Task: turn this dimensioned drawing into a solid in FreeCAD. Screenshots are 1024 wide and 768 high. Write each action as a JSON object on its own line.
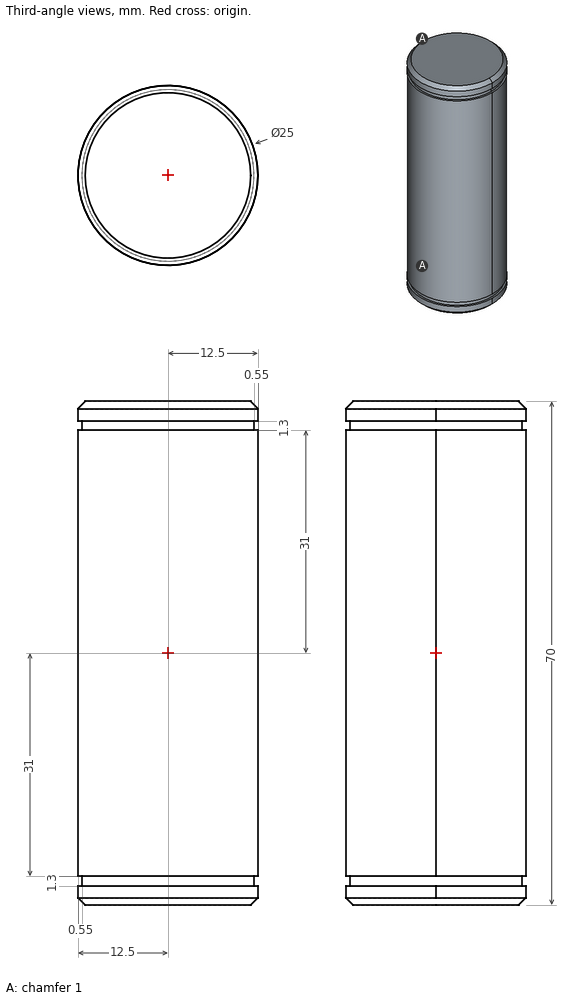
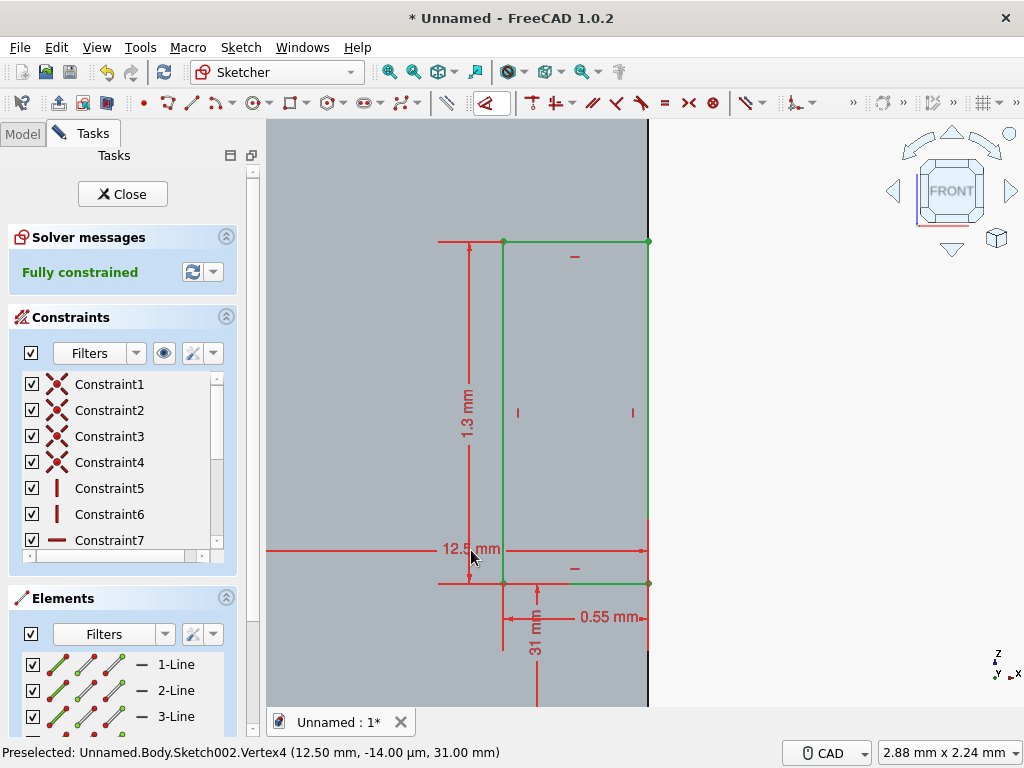
{"action": "left_click", "coordinate": [123, 194]}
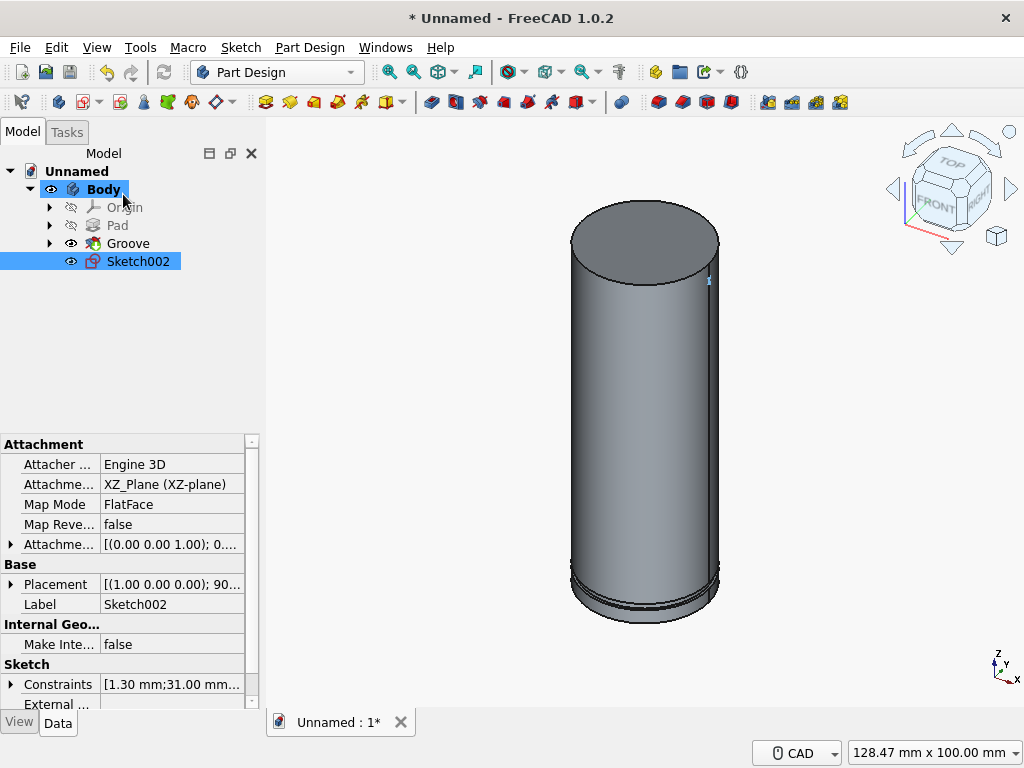
{"action": "left_click", "coordinate": [480, 102]}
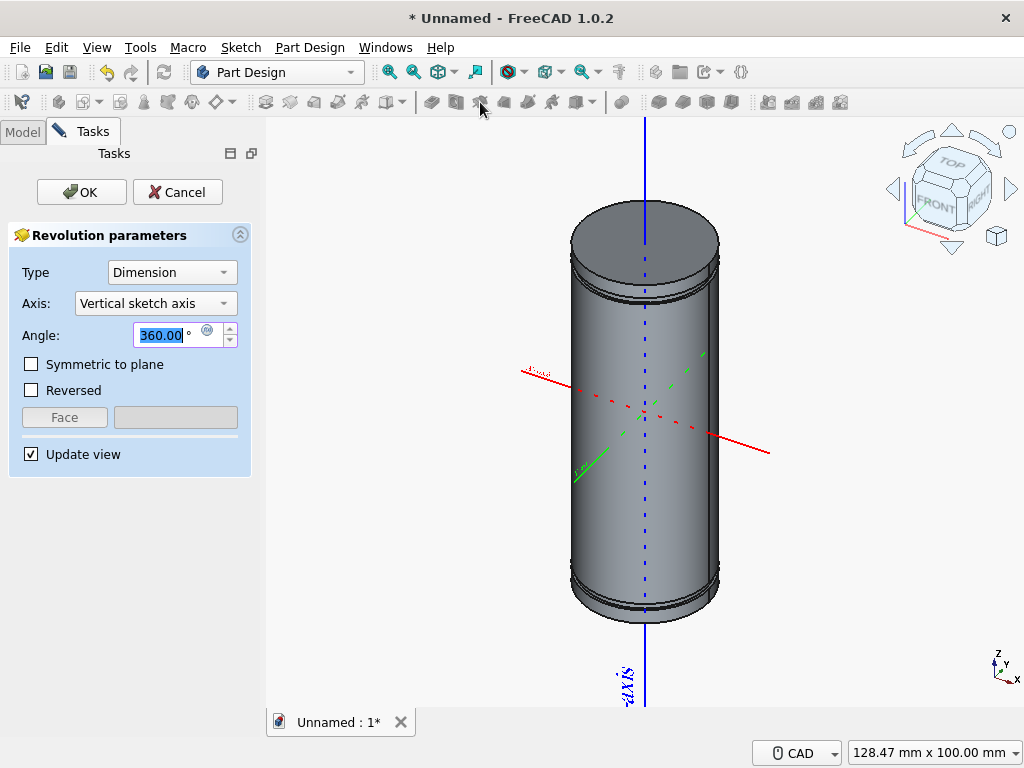
{"action": "left_click", "coordinate": [82, 192]}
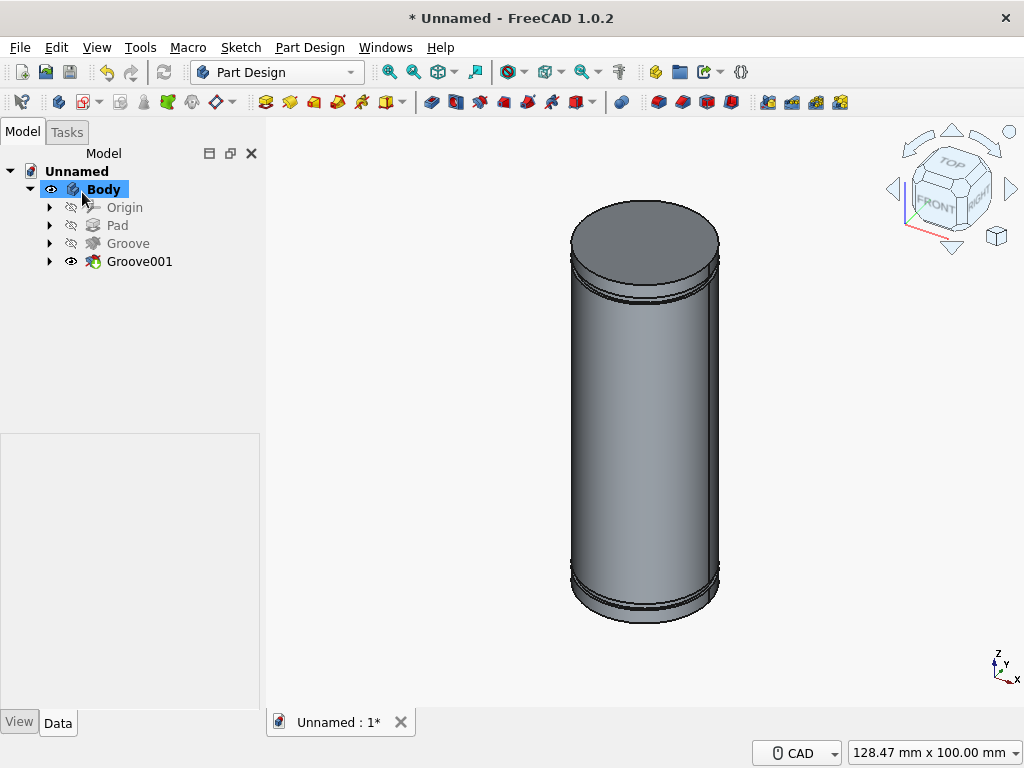
{"action": "left_click", "coordinate": [572, 246]}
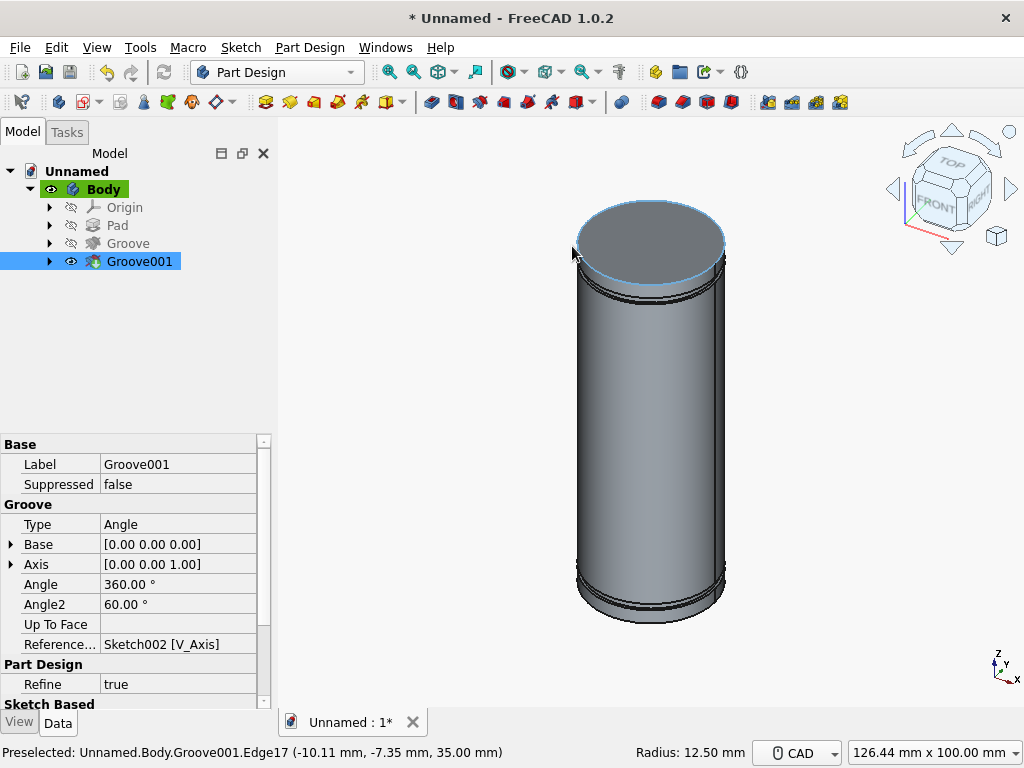
{"action": "key", "text": "0"}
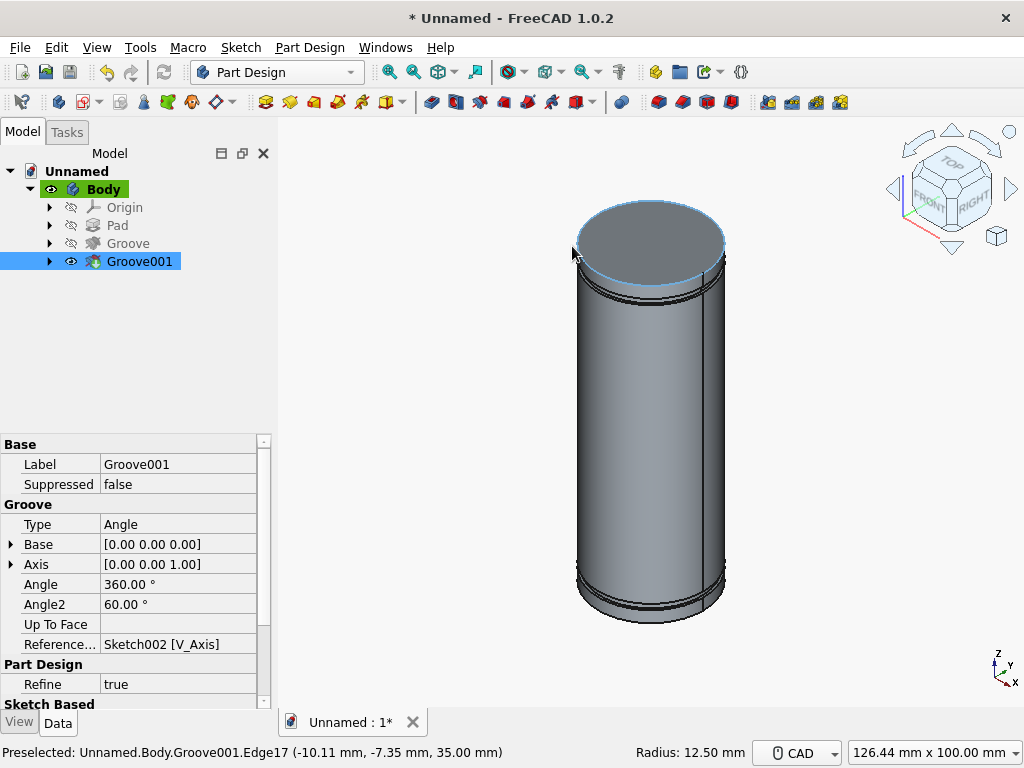
{"action": "key", "text": "2"}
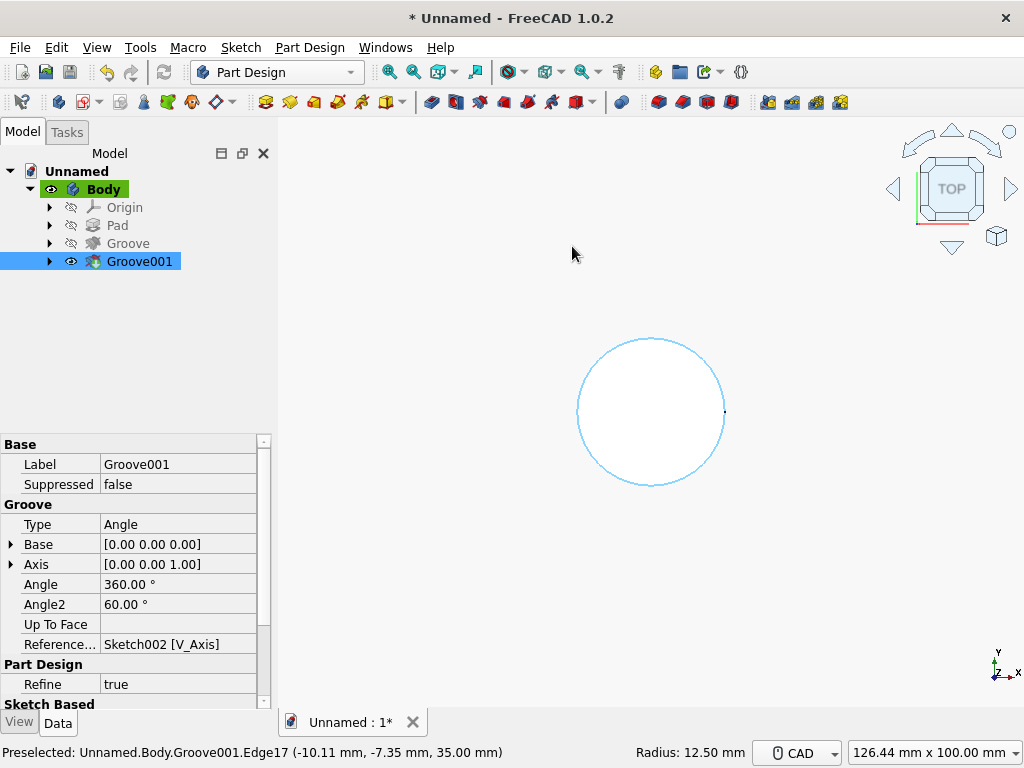
{"action": "key", "text": "v f"}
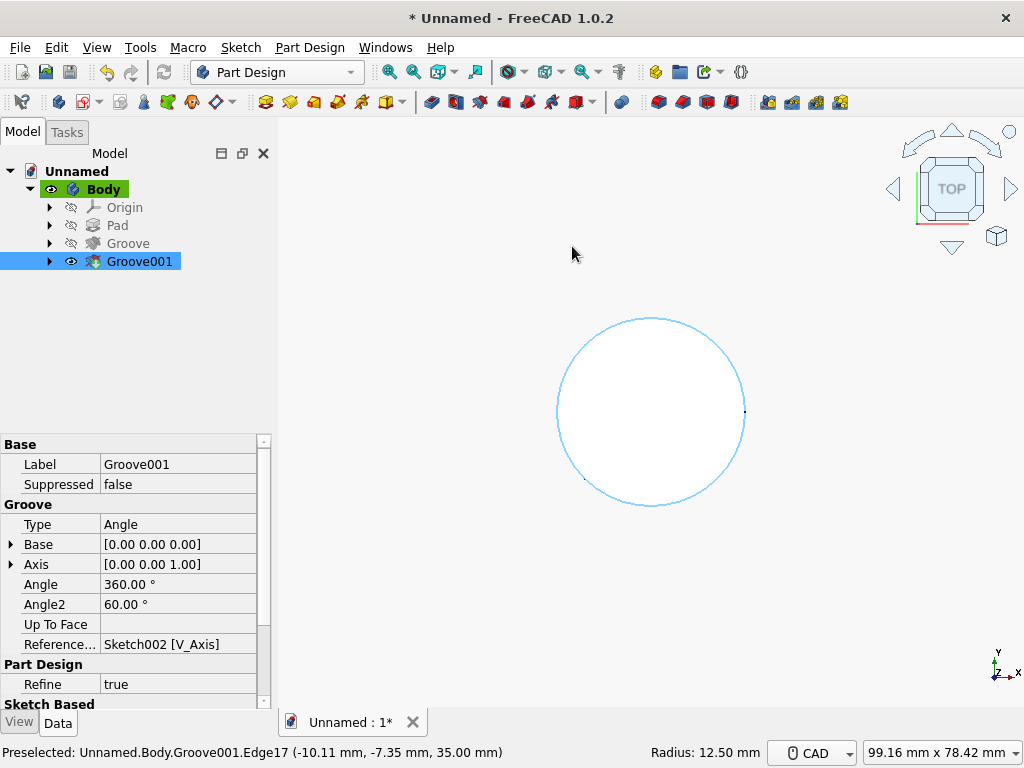
{"action": "key", "text": "1"}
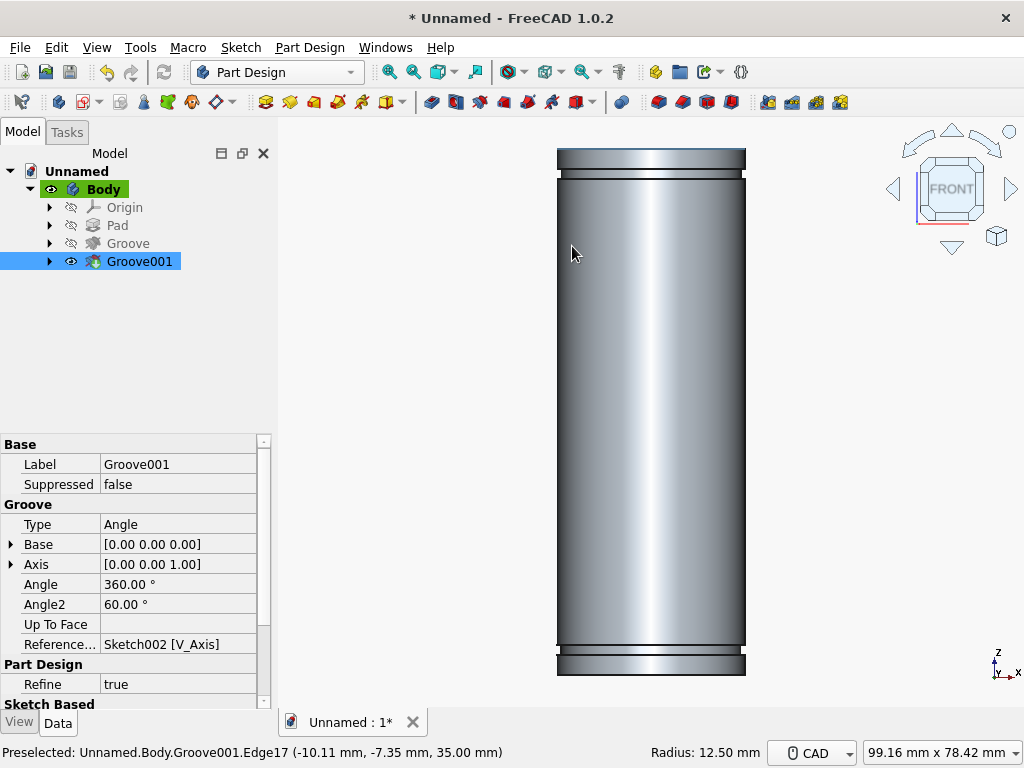
{"action": "left_click", "coordinate": [575, 674], "text": "ctrl"}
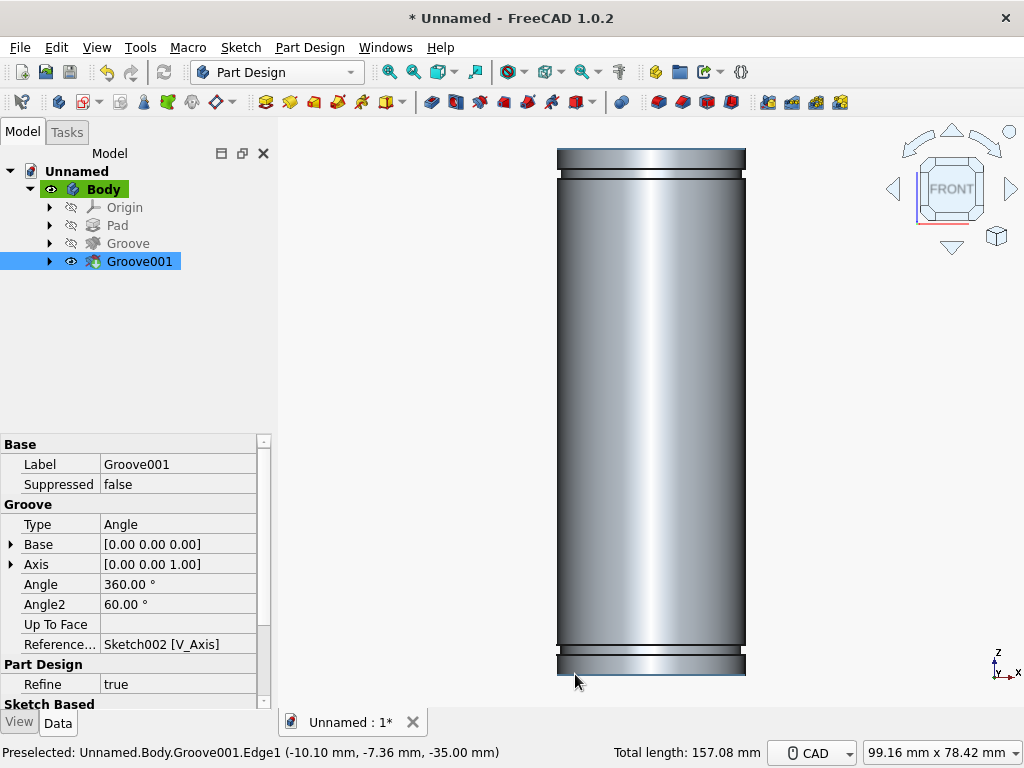
{"action": "left_click", "coordinate": [684, 102]}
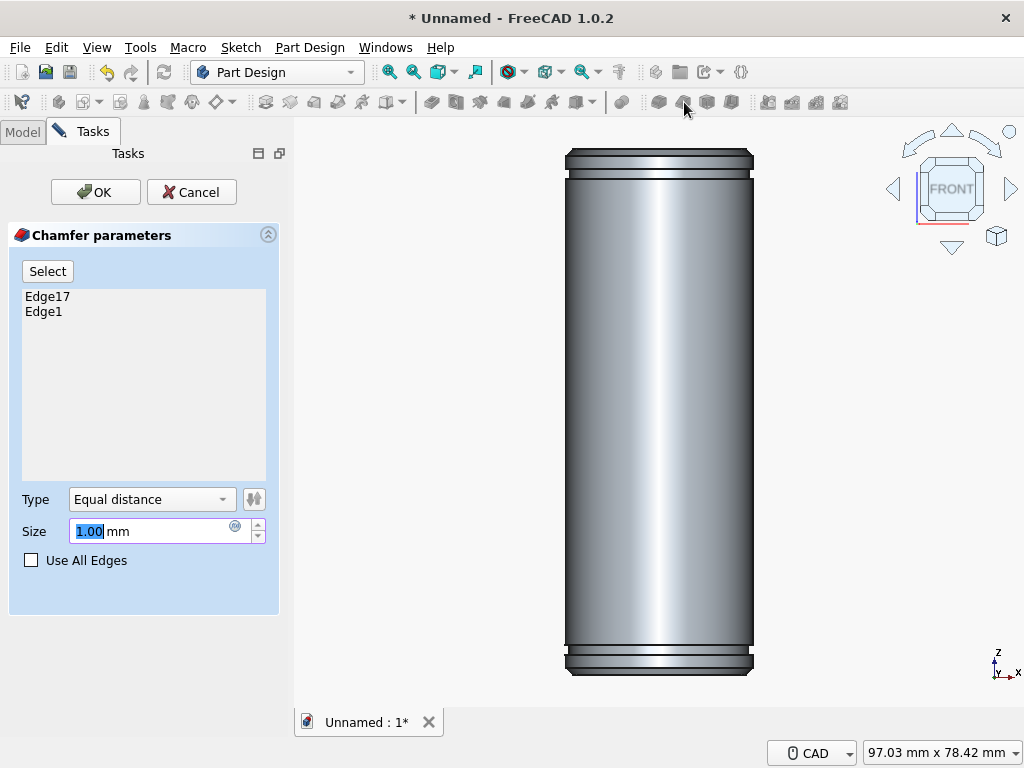
{"action": "type", "text": "1"}
{"action": "key", "text": "Tab"}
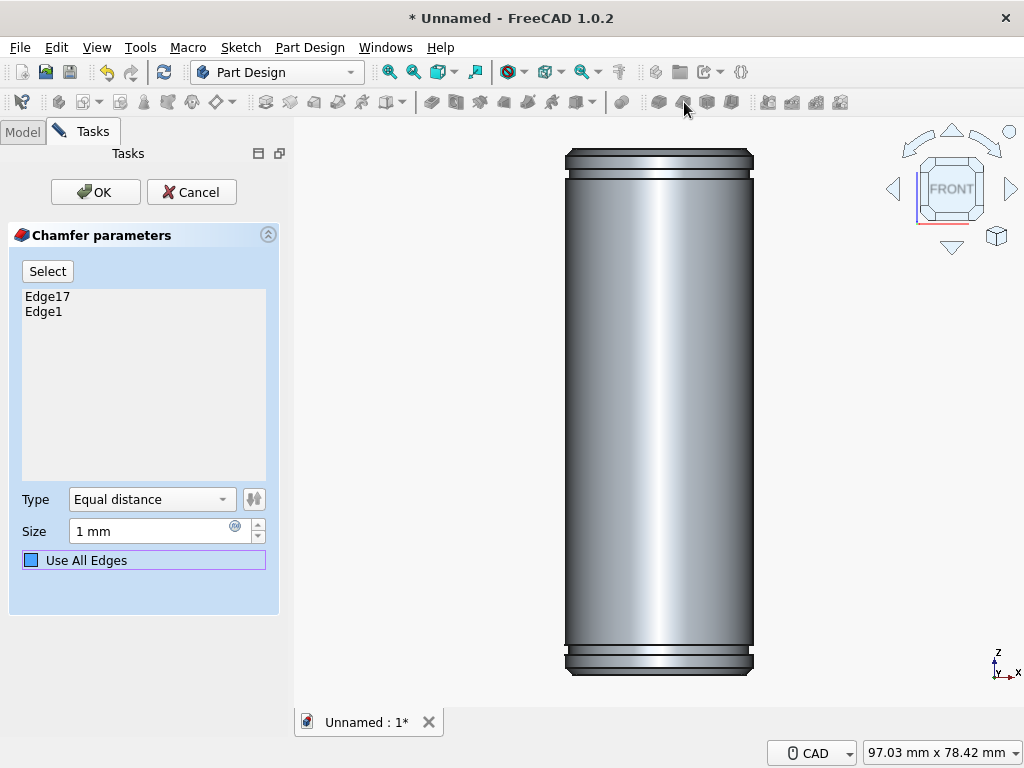
{"action": "left_click", "coordinate": [96, 192]}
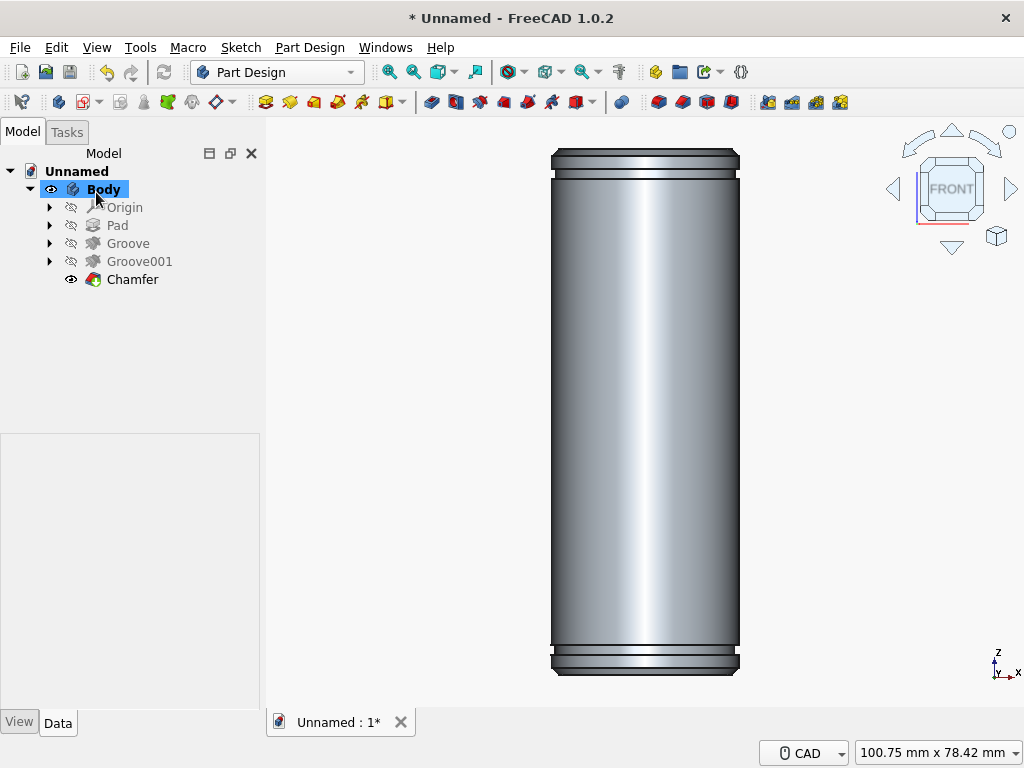
{"action": "key", "text": "0"}